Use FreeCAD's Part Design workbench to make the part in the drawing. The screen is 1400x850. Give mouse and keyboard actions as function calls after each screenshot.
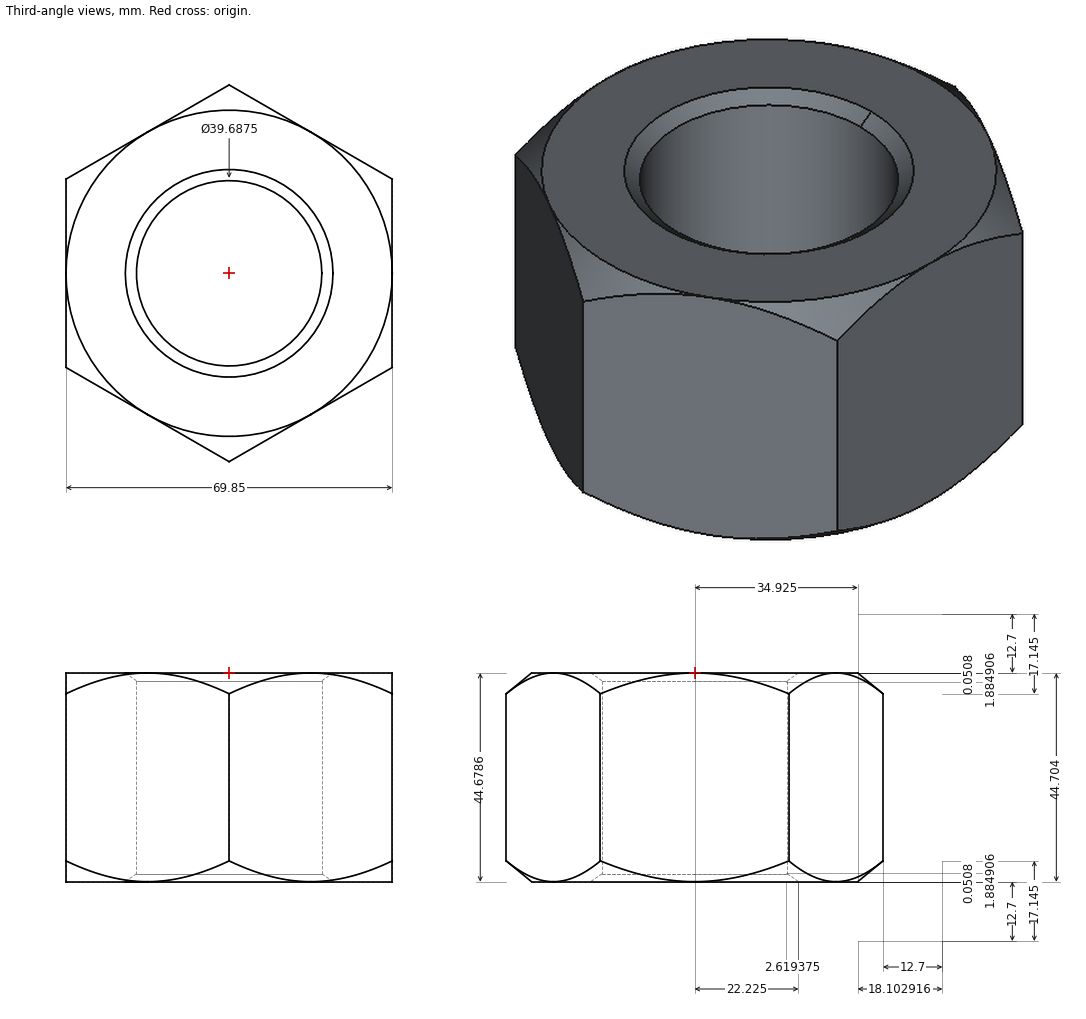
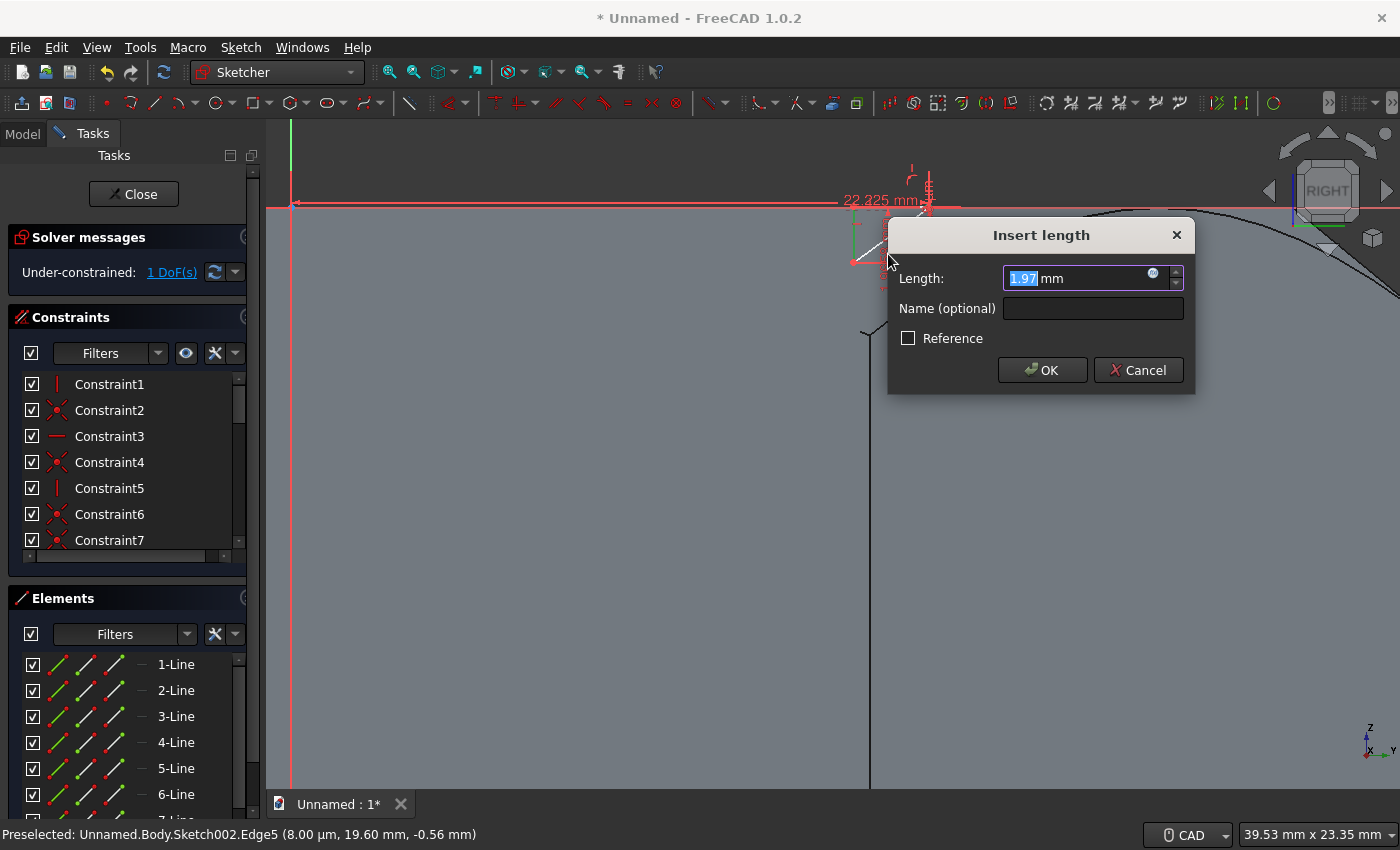
text(1.884906)
key(Return)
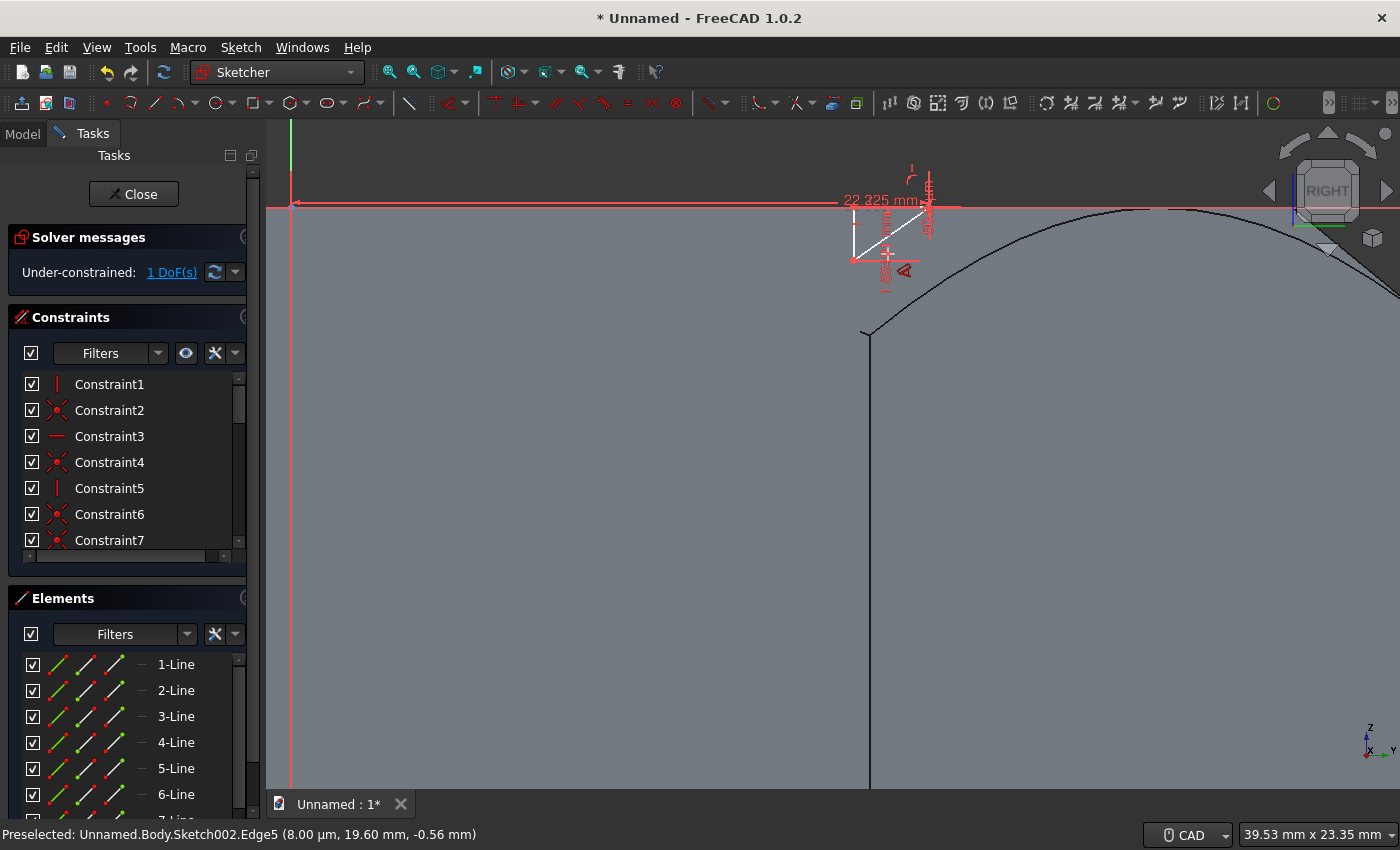
click(906, 207)
click(891, 173)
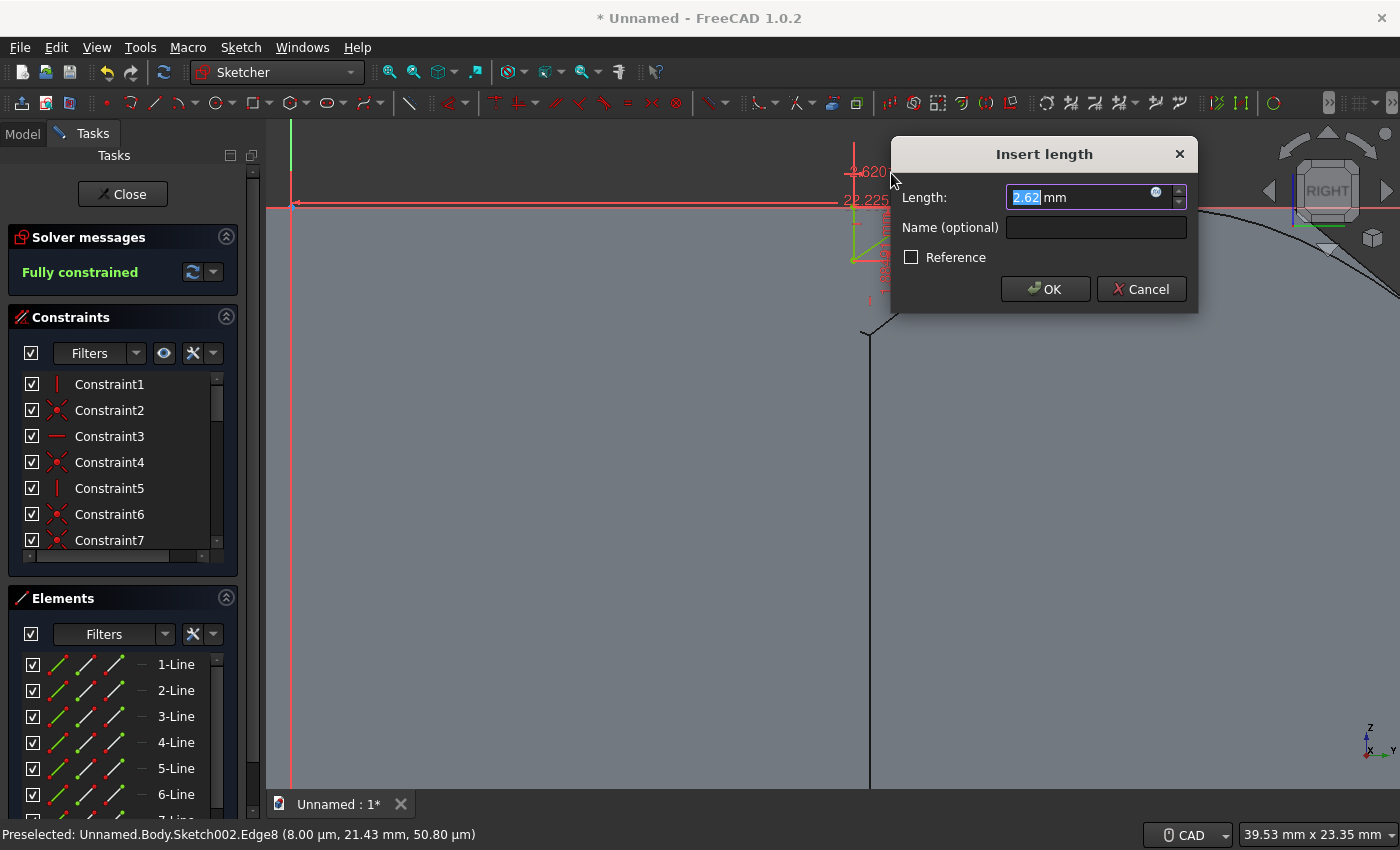
text(2.619375)
key(Return)
key(Escape)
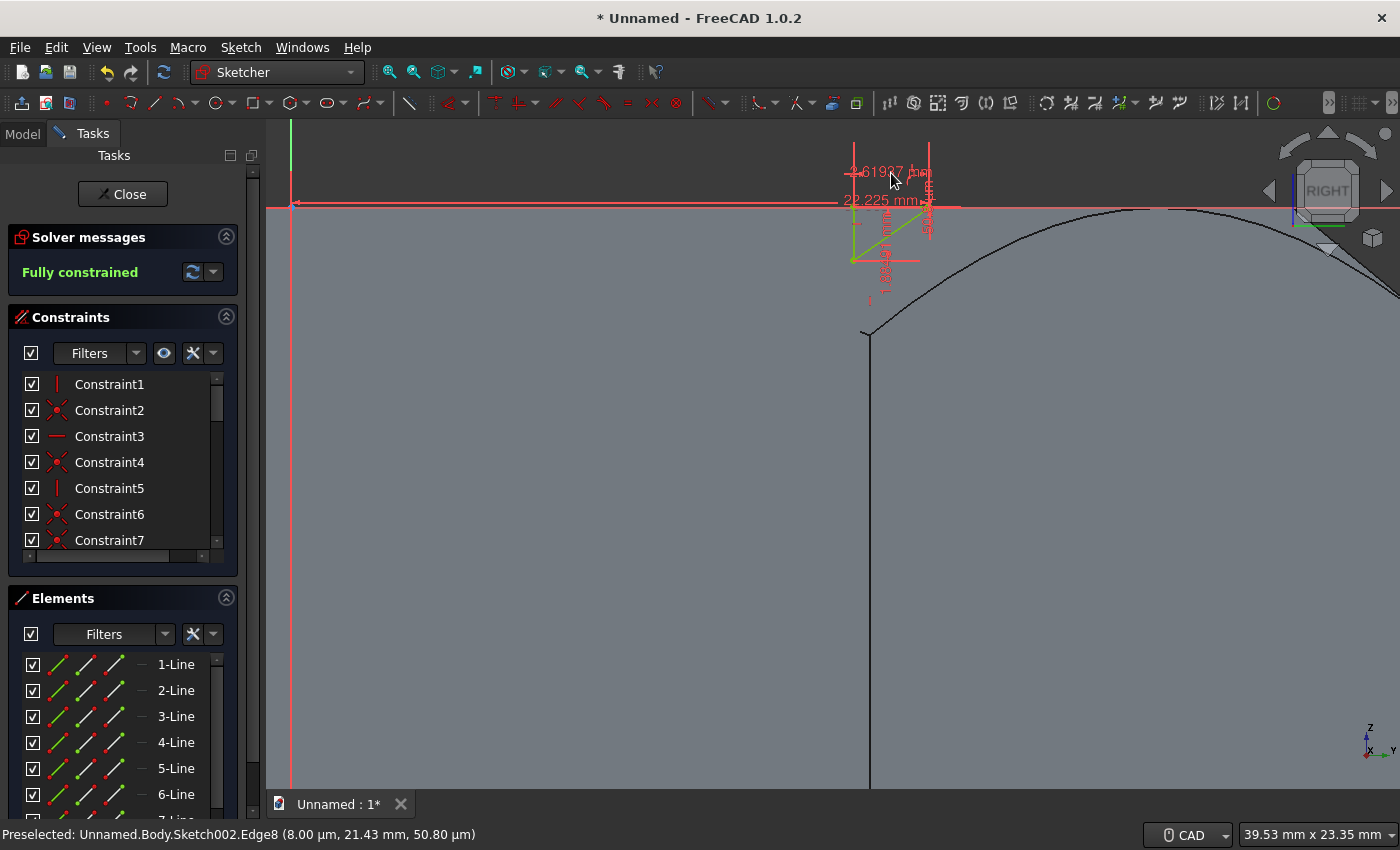
click(123, 194)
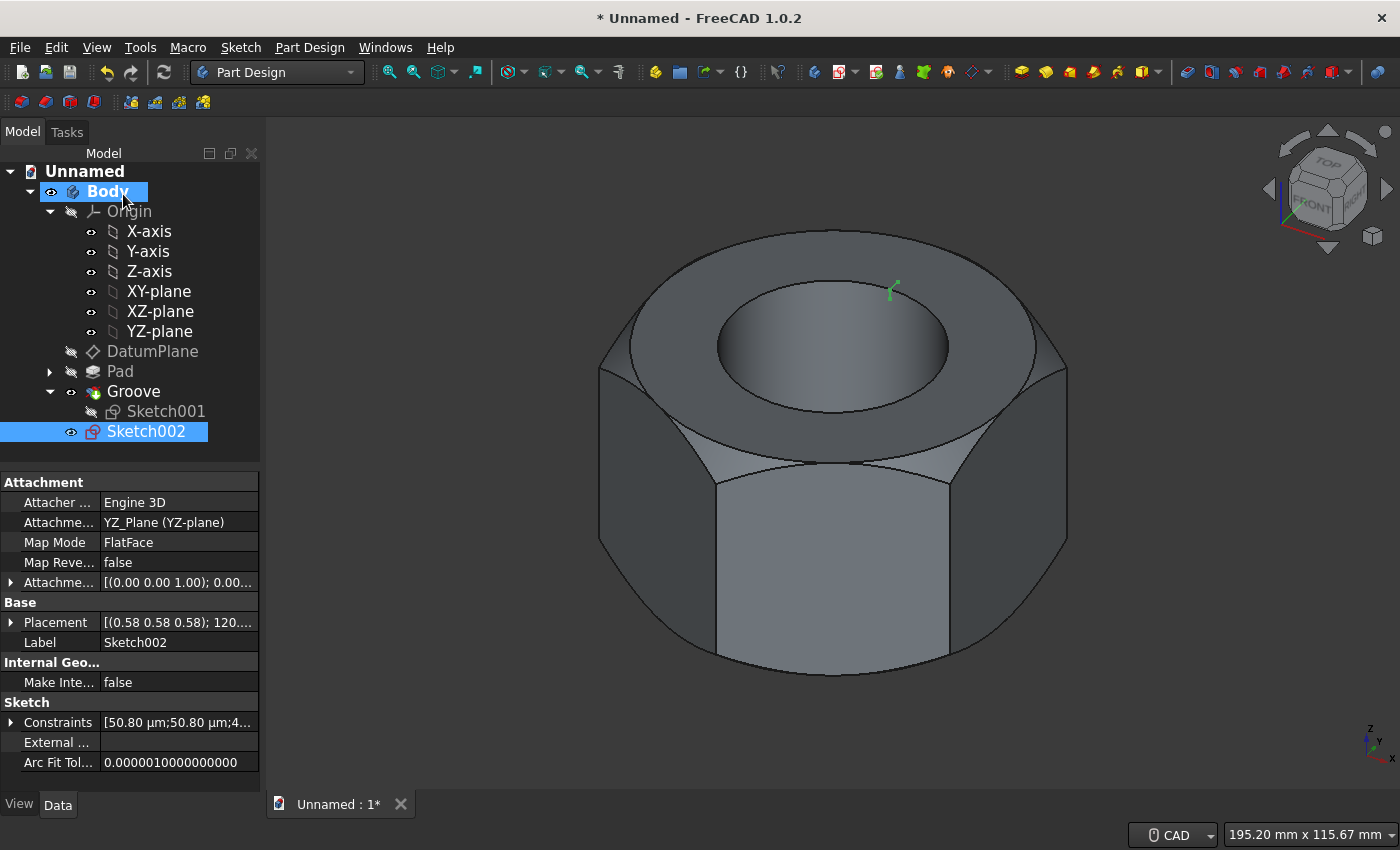
click(1236, 72)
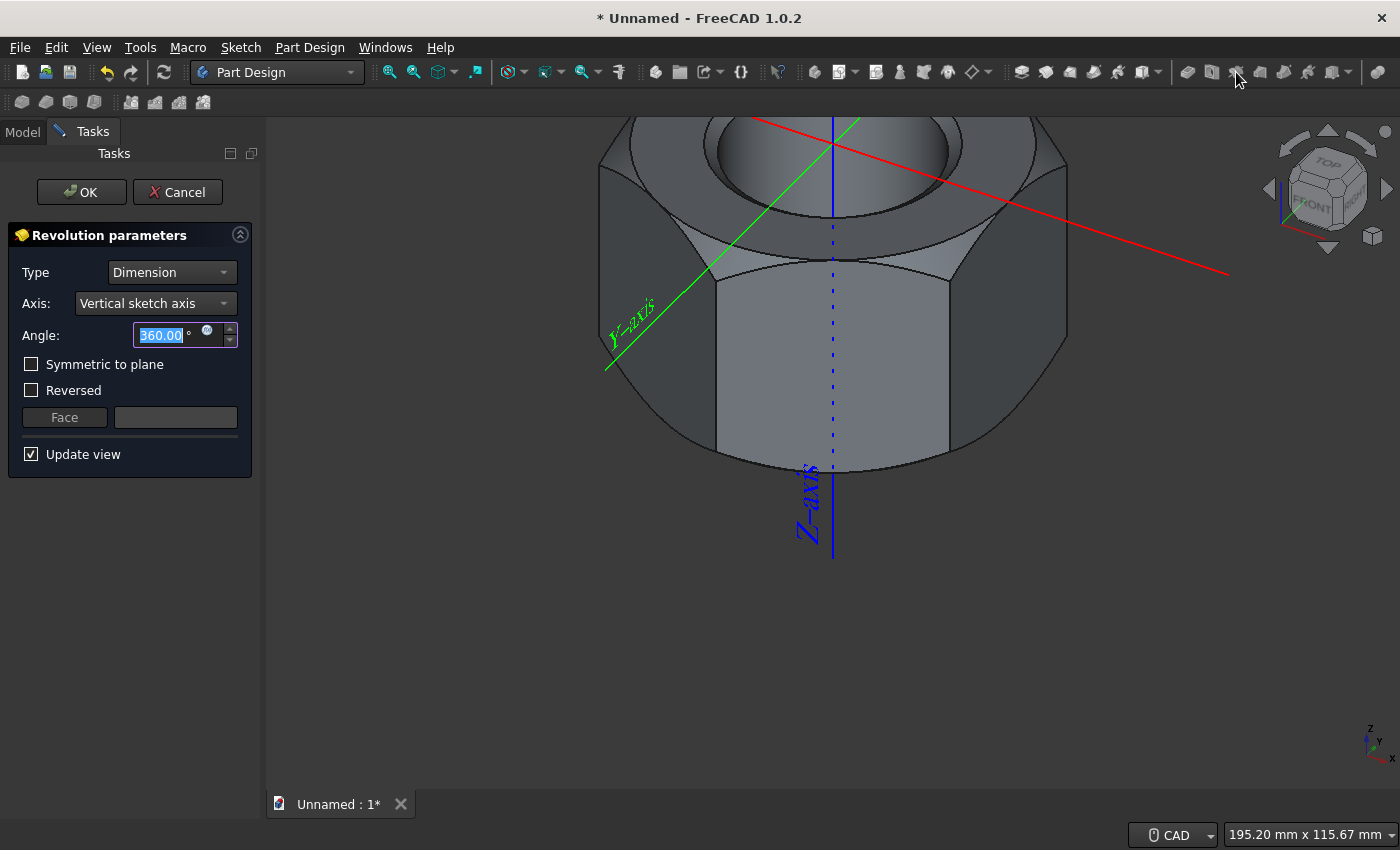
click(82, 192)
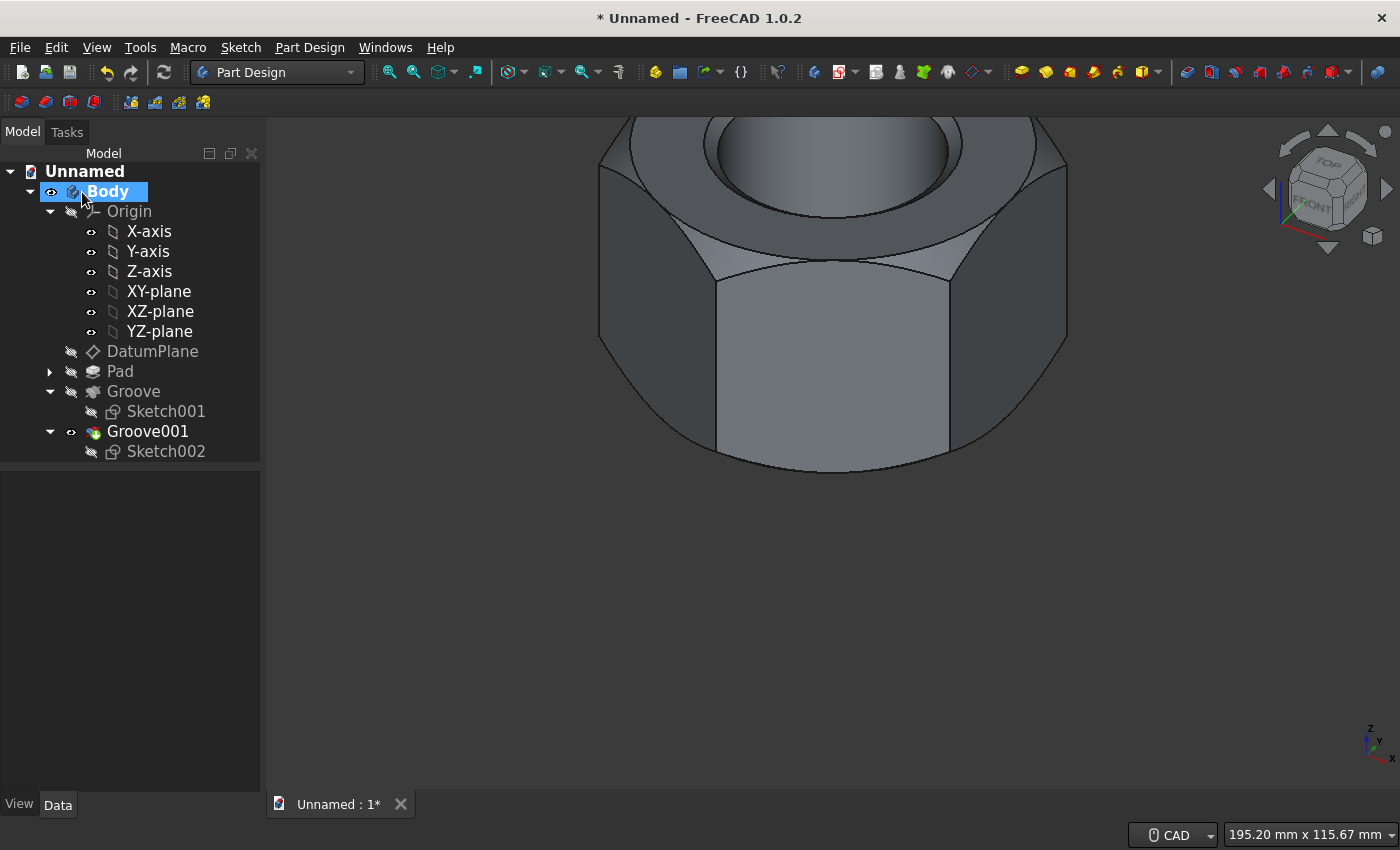
key(0)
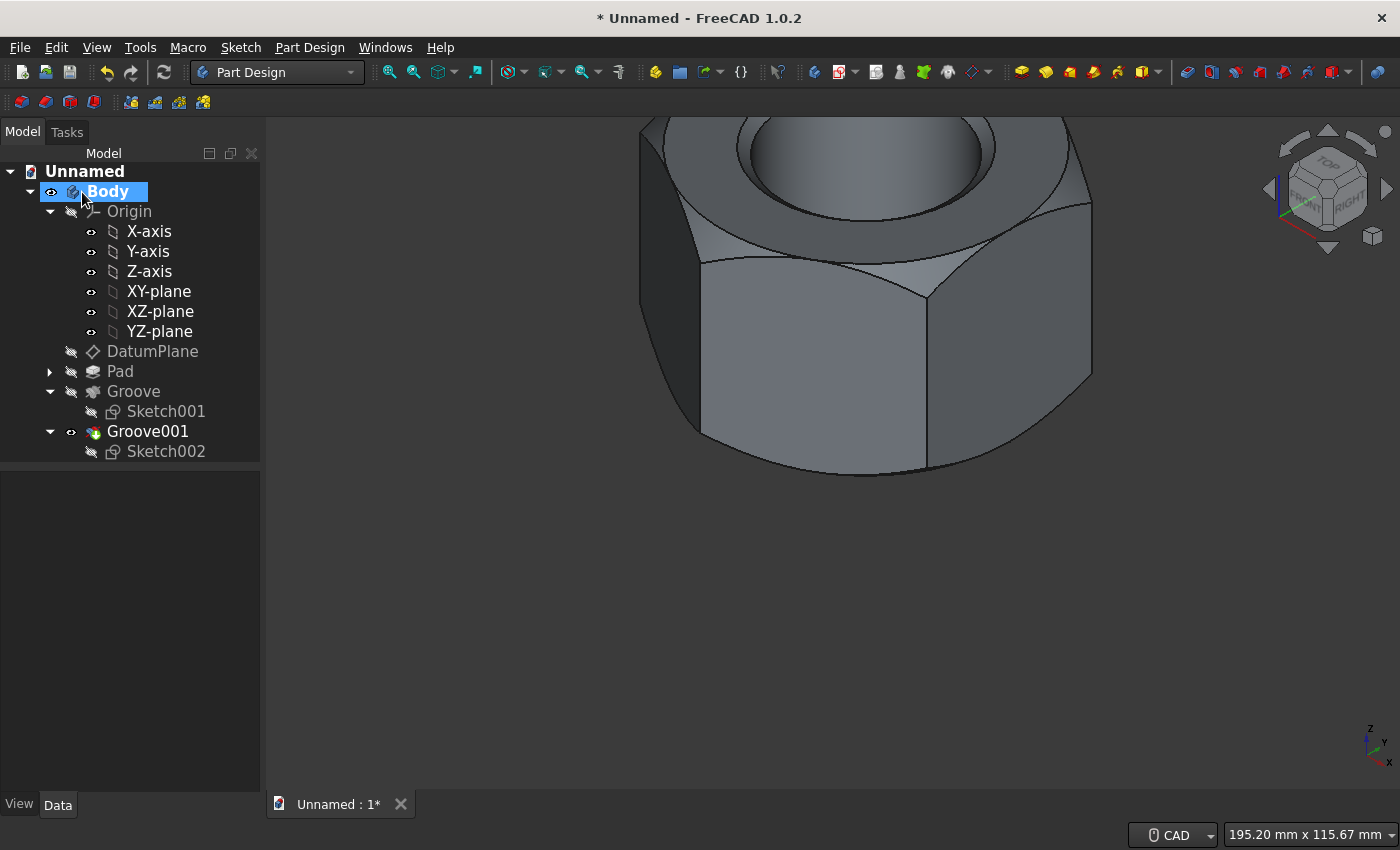
key(v)
key(f)